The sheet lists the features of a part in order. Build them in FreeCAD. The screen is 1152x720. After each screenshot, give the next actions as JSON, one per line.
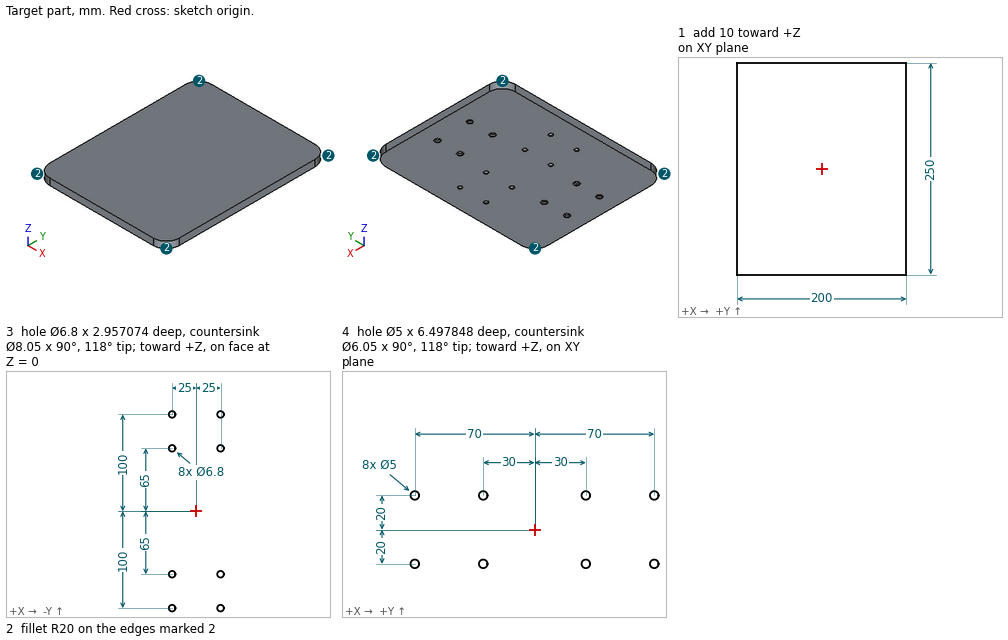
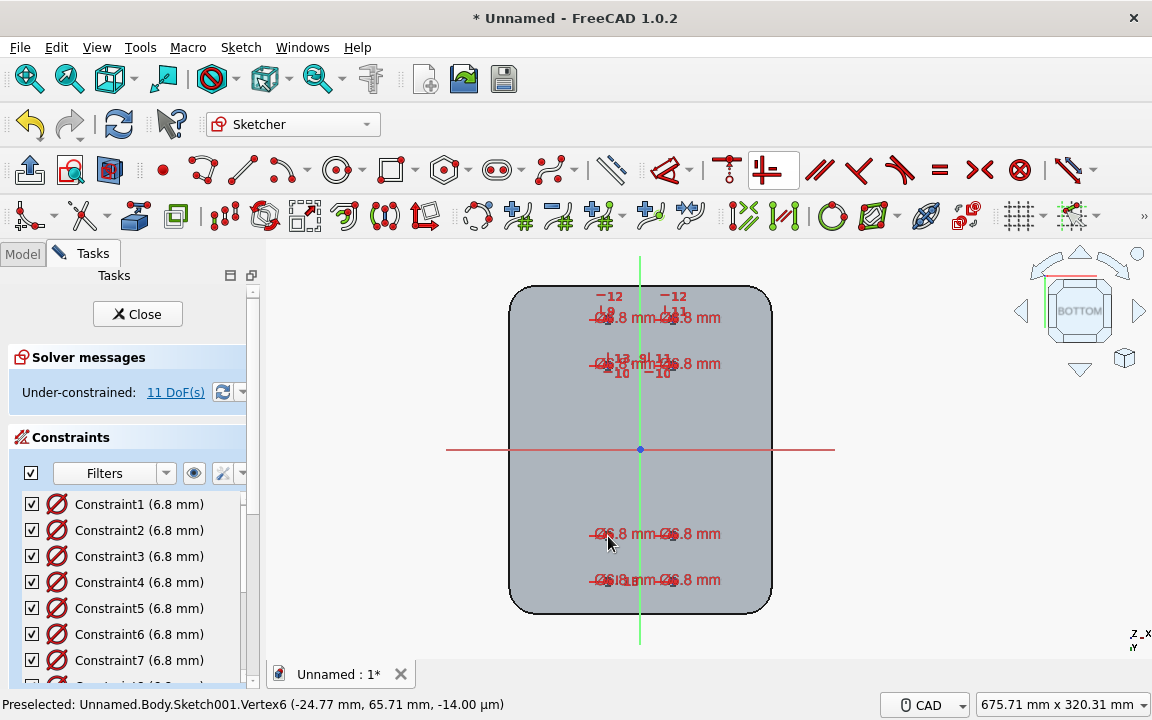
{"action": "key", "text": "v"}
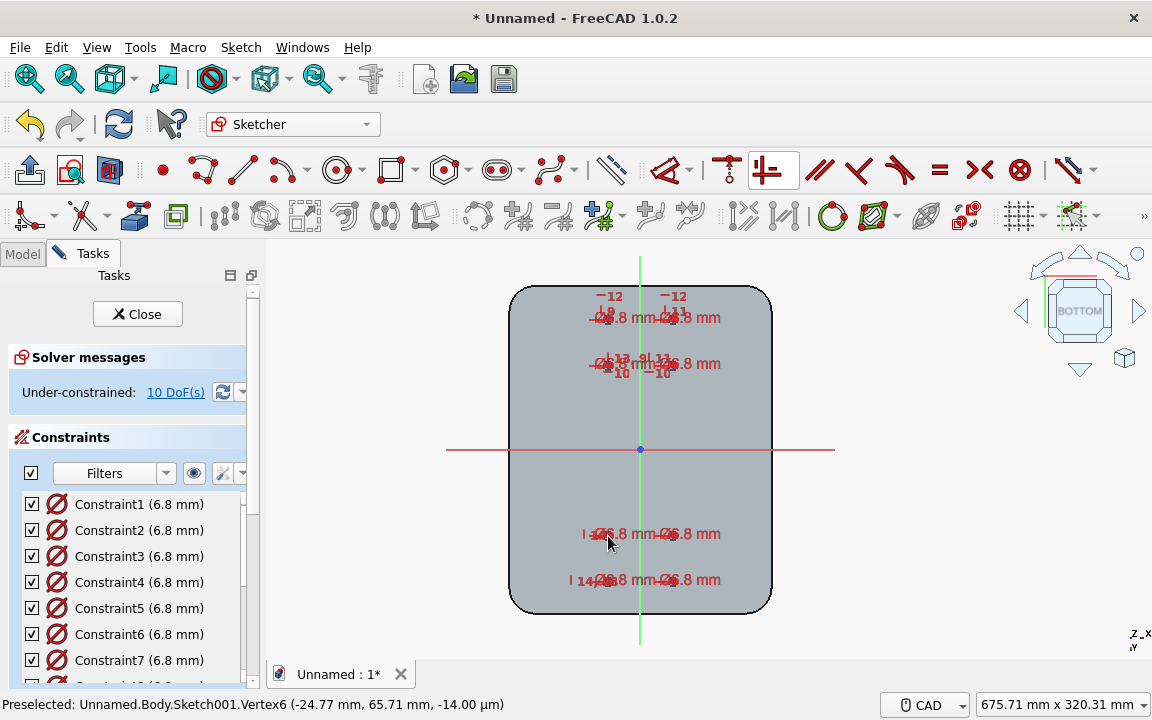
{"action": "left_click", "coordinate": [673, 366]}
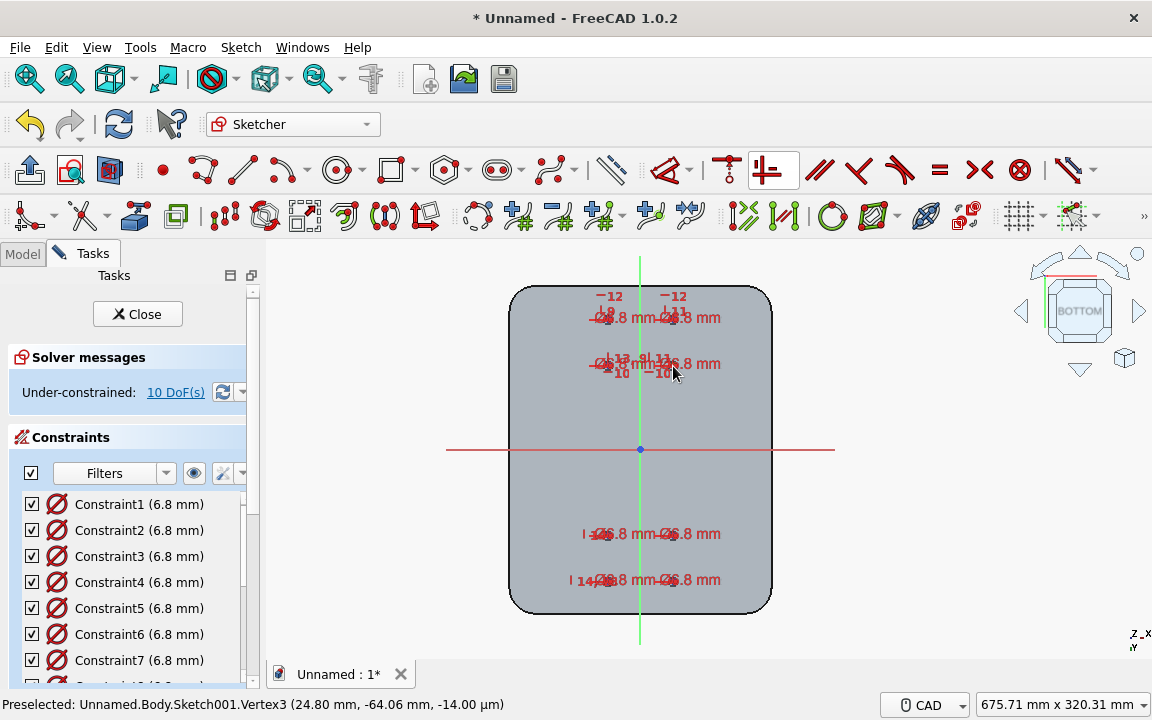
{"action": "left_click", "coordinate": [673, 536]}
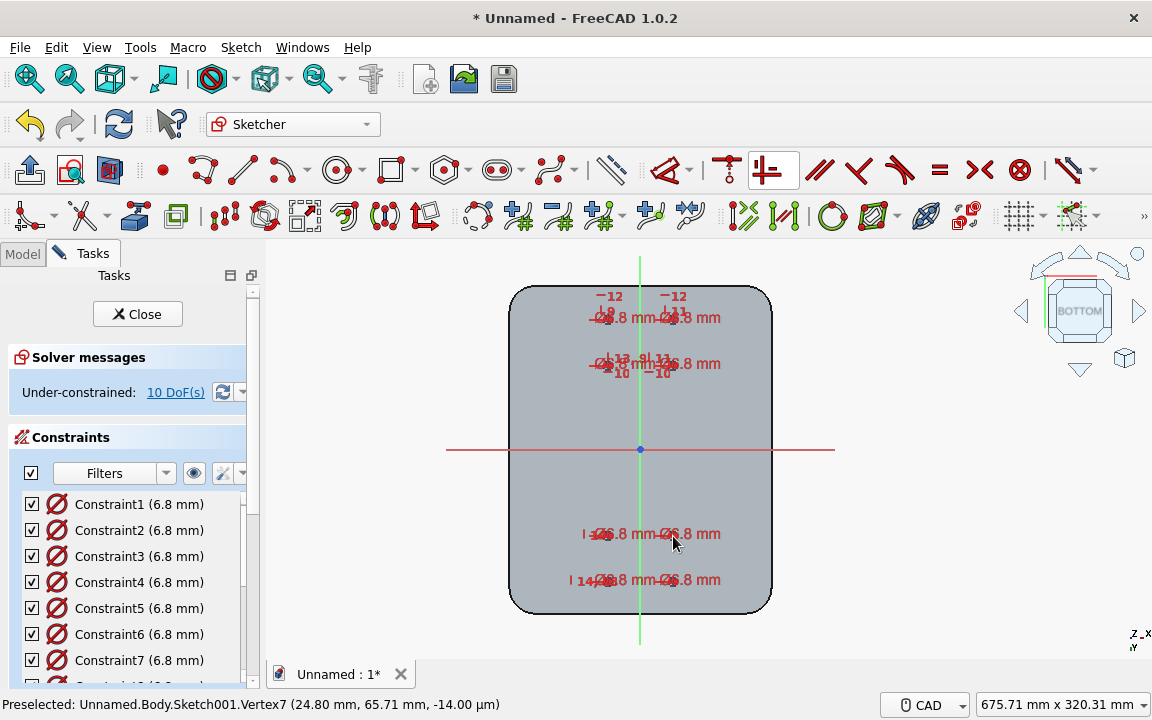
{"action": "key", "text": "v"}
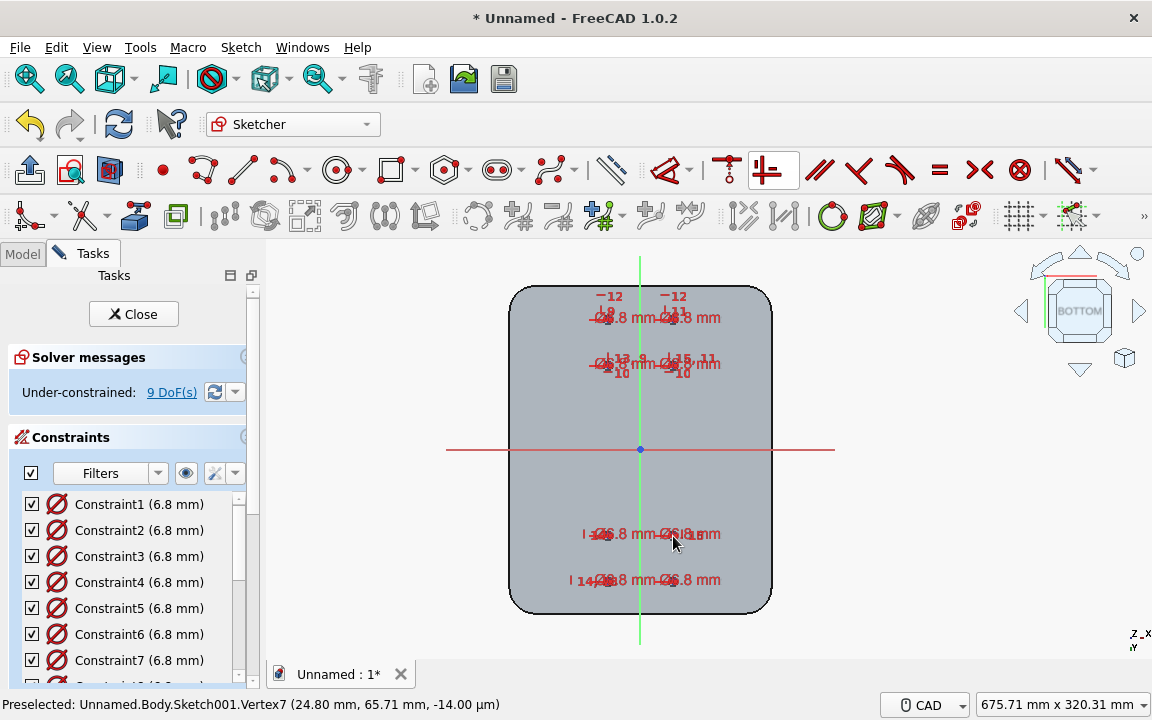
{"action": "left_click", "coordinate": [608, 536]}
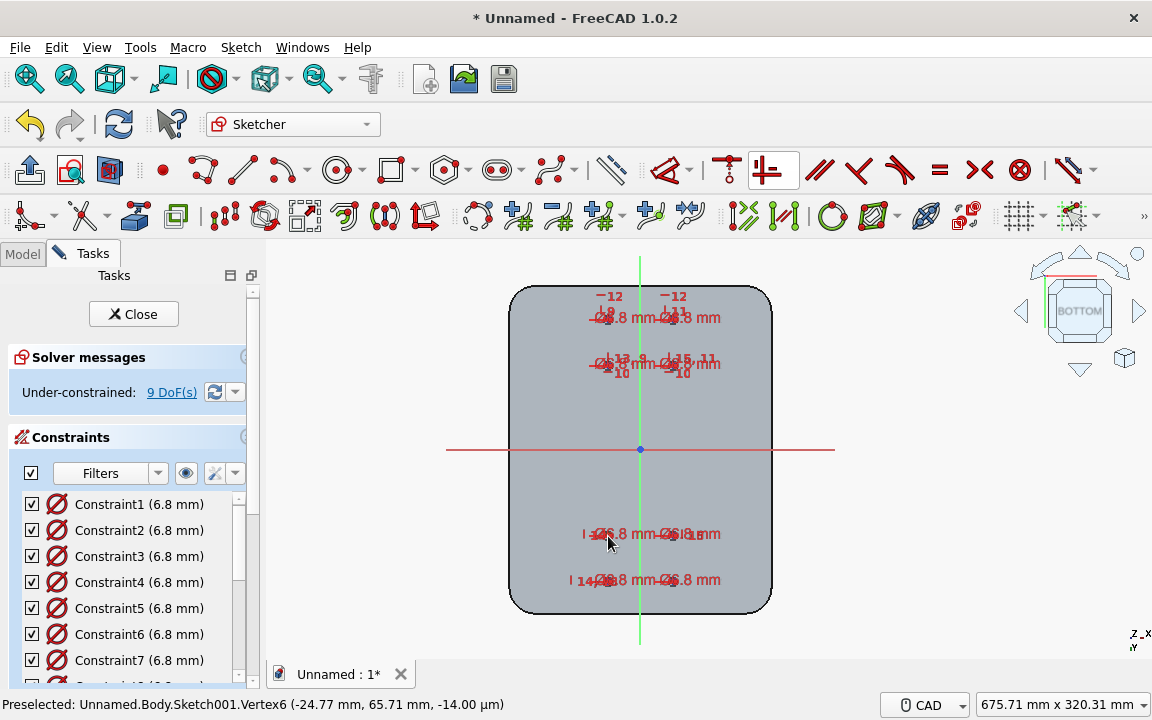
{"action": "left_click", "coordinate": [673, 536]}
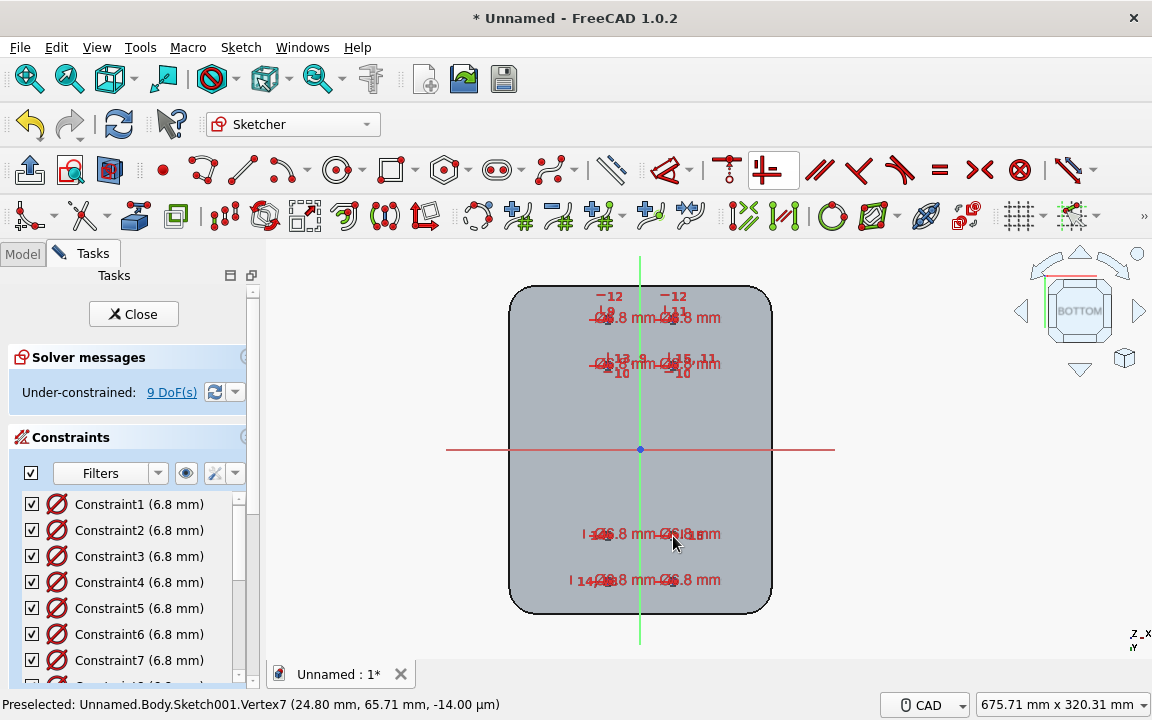
{"action": "key", "text": "h"}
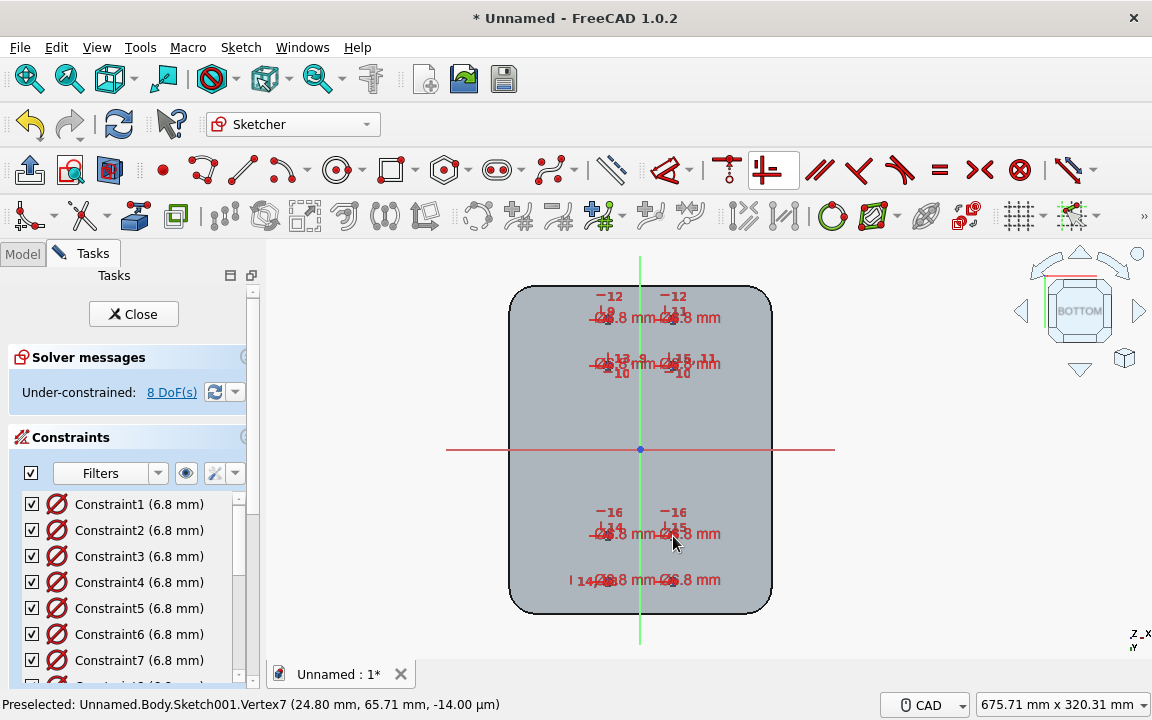
{"action": "left_click", "coordinate": [673, 536]}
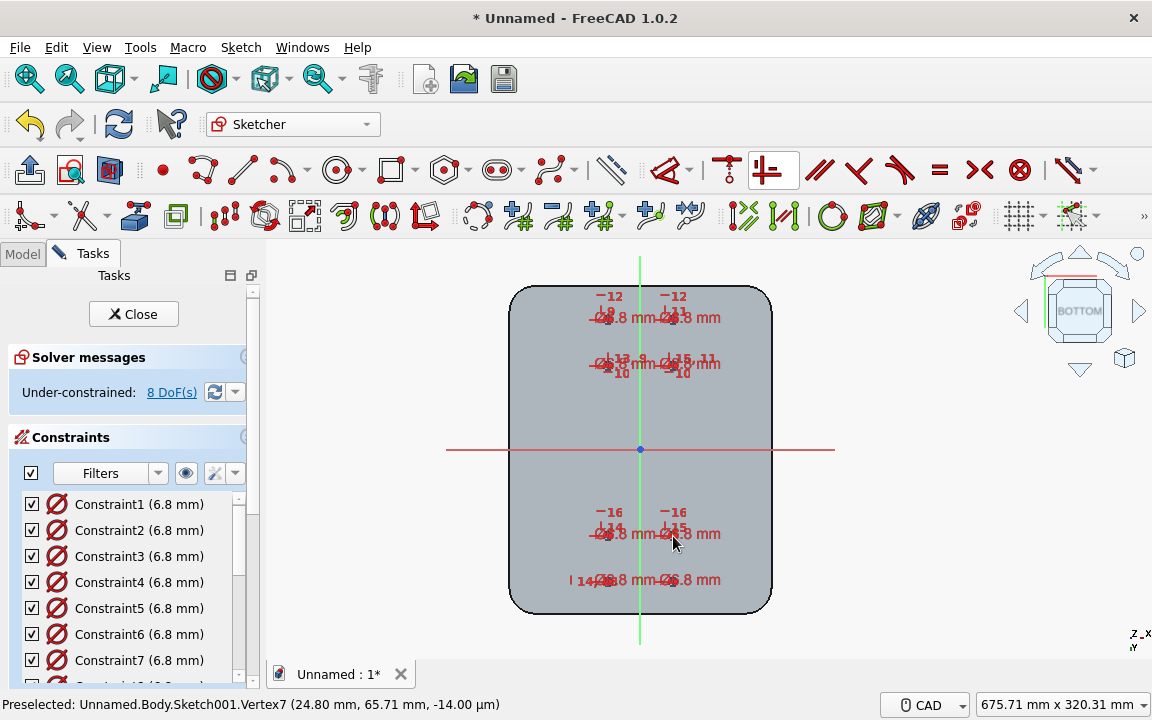
{"action": "left_click", "coordinate": [673, 582]}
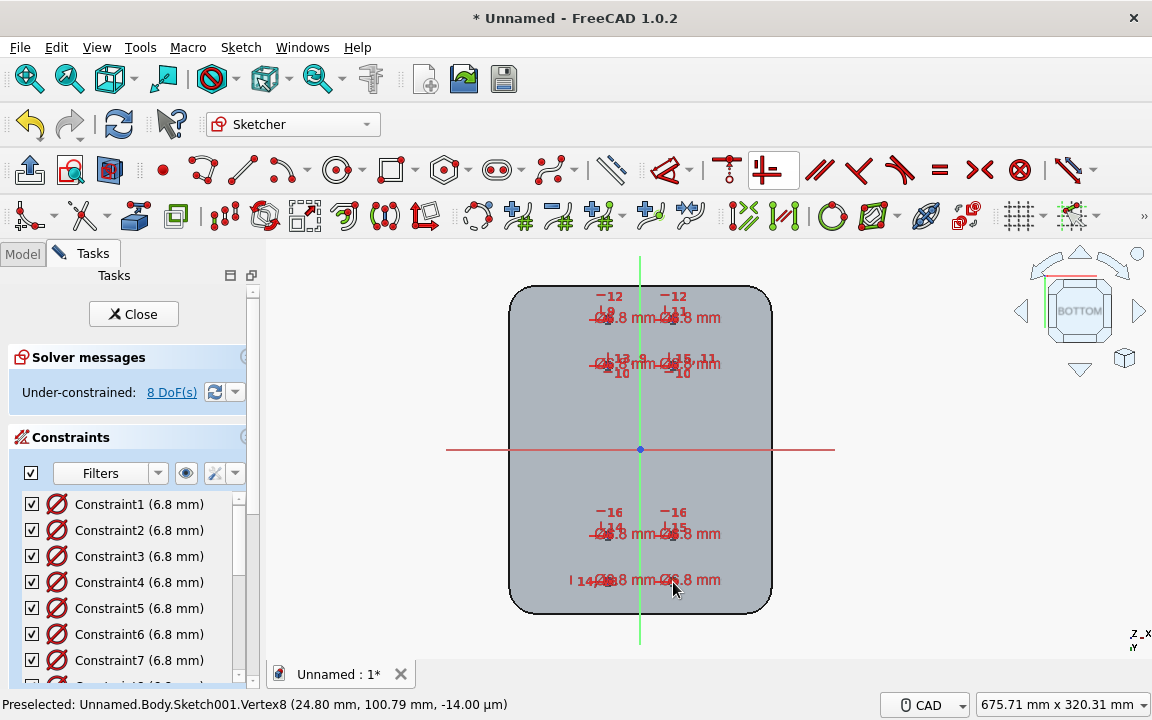
{"action": "key", "text": "v"}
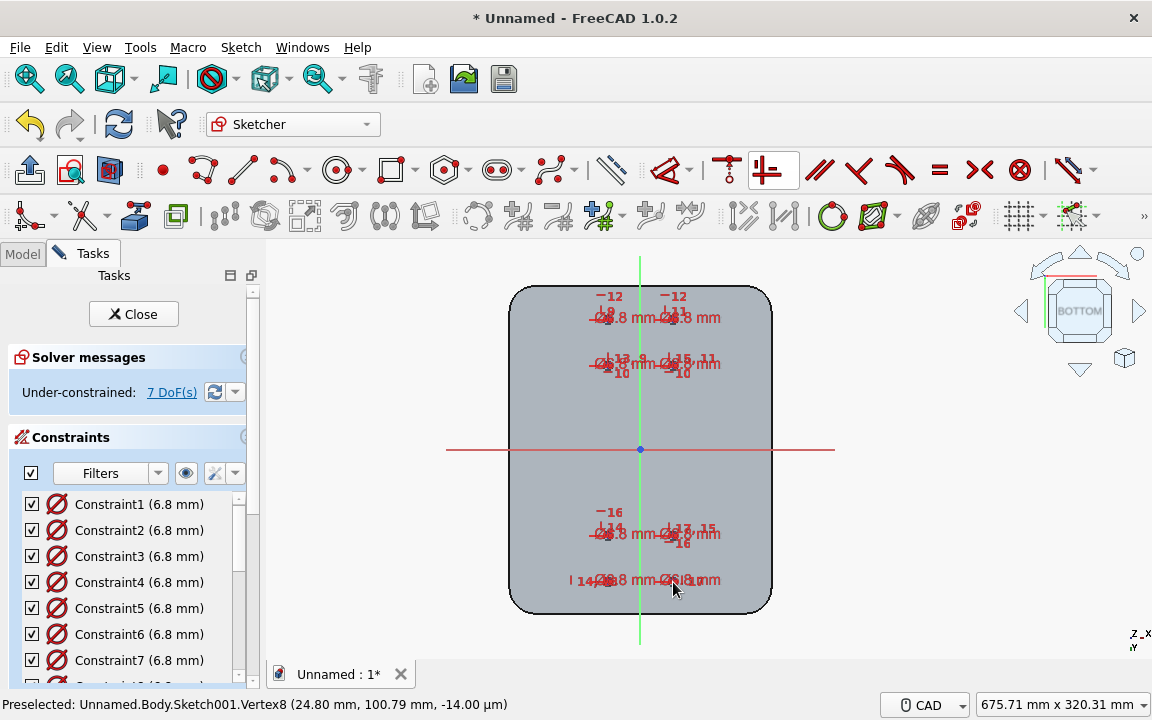
{"action": "left_click", "coordinate": [608, 582]}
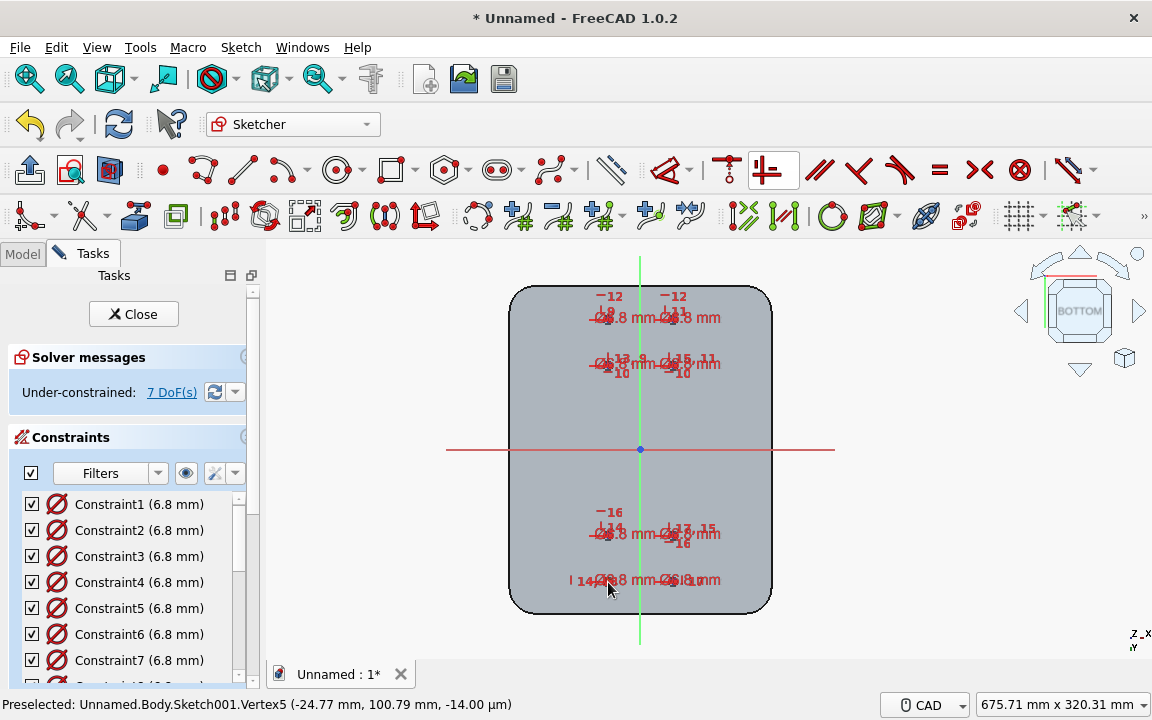
{"action": "left_click", "coordinate": [673, 582]}